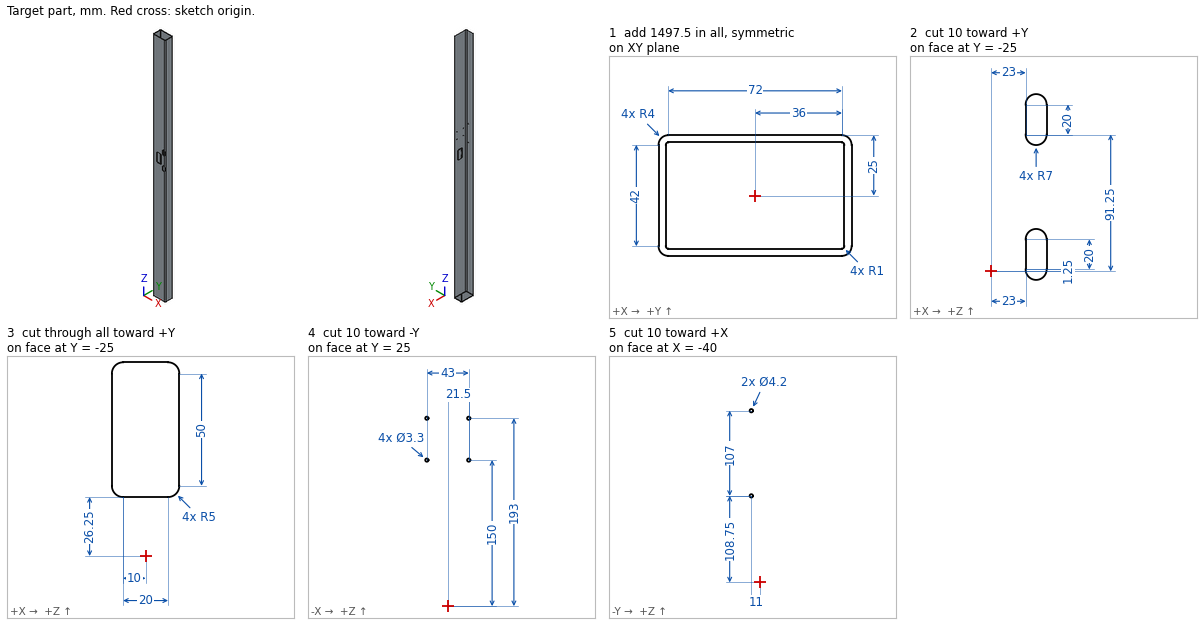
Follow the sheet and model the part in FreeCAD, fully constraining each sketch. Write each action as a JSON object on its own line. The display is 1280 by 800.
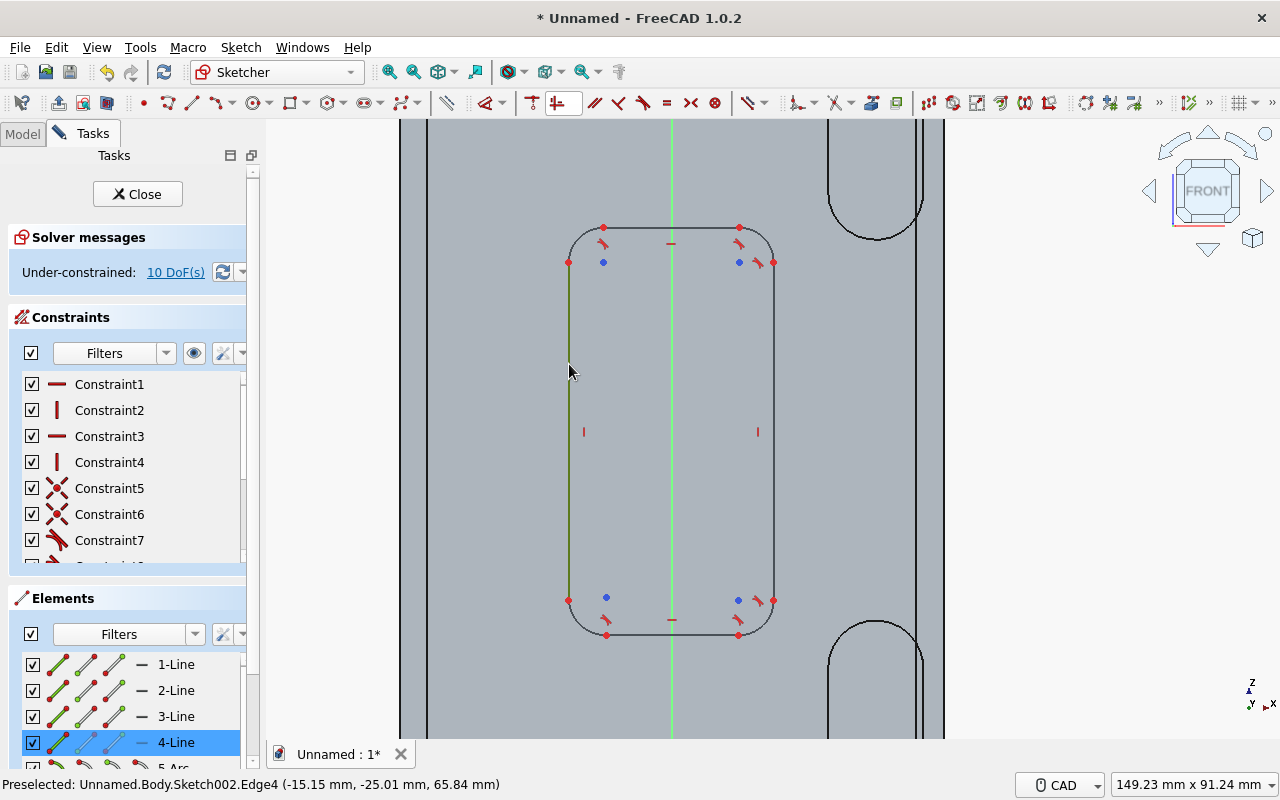
{"action": "left_click", "coordinate": [588, 232]}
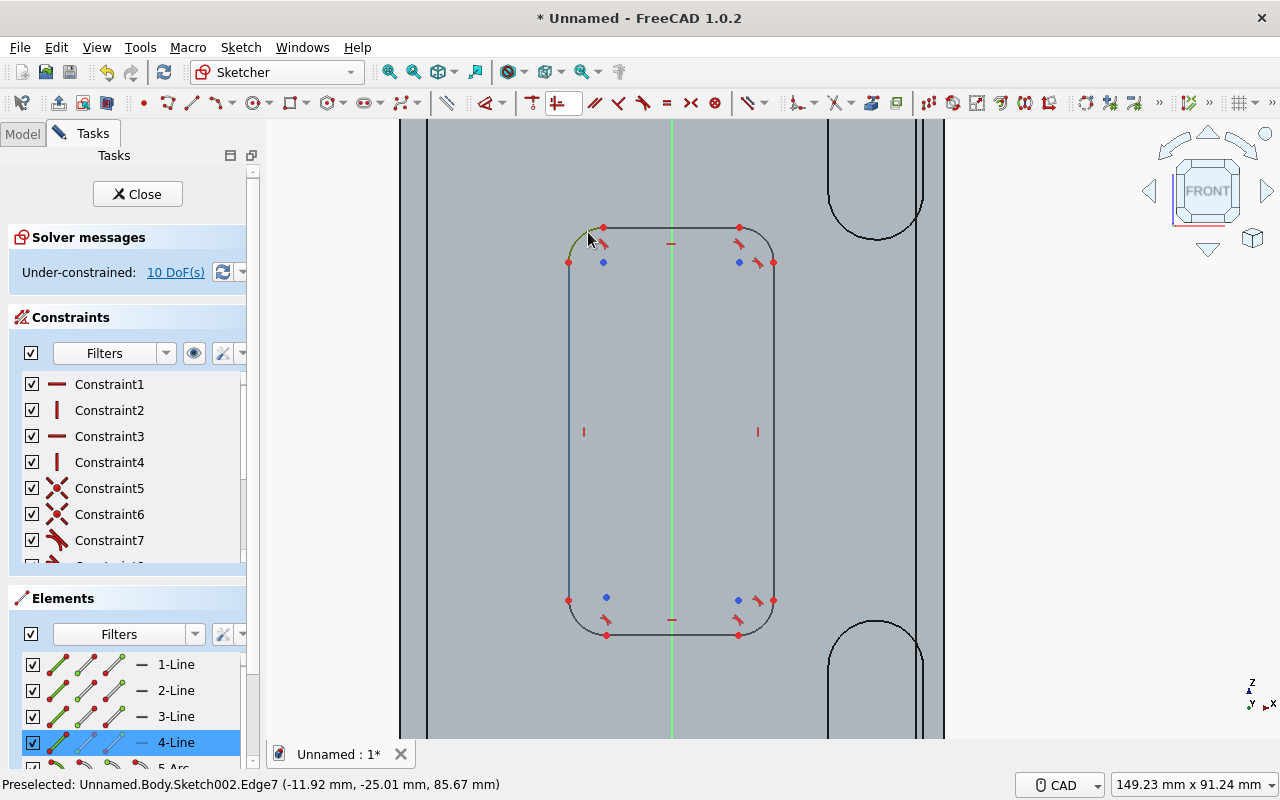
{"action": "key", "text": "t"}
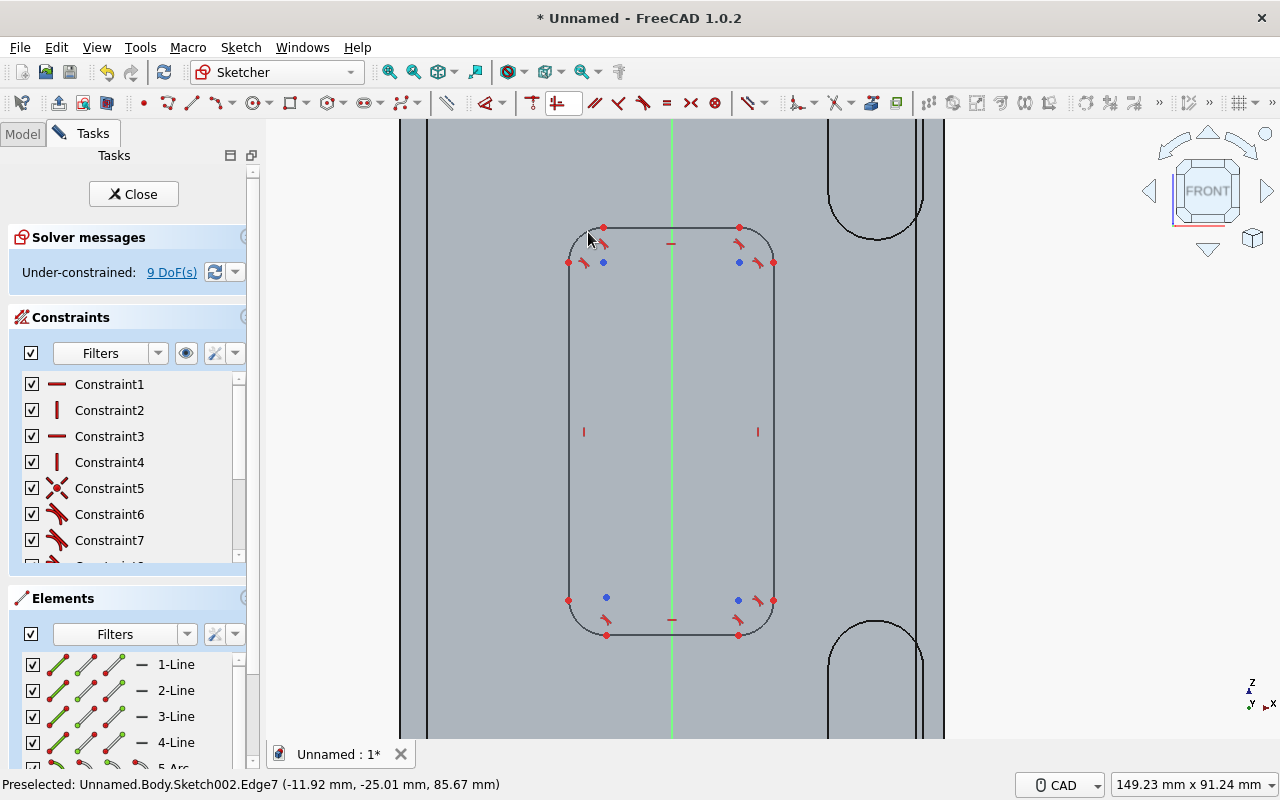
{"action": "left_click", "coordinate": [569, 364]}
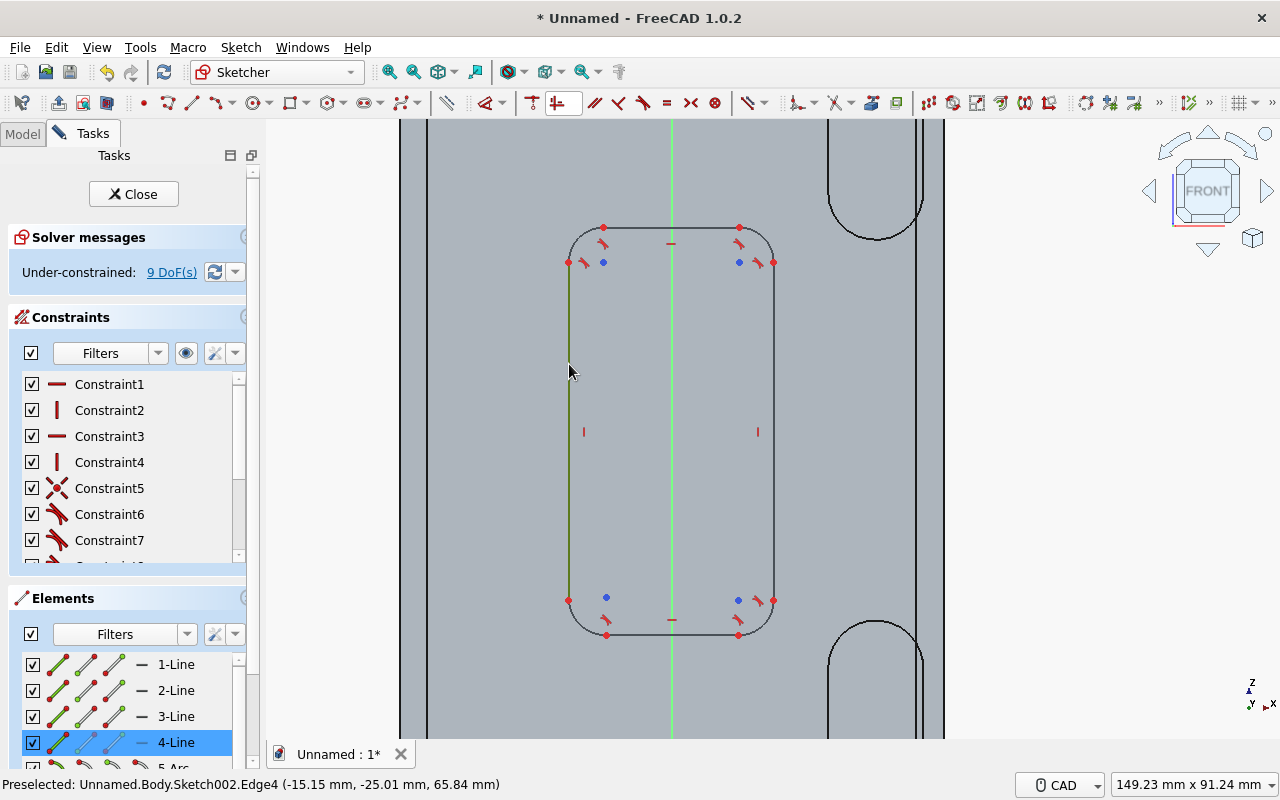
{"action": "left_click", "coordinate": [574, 617]}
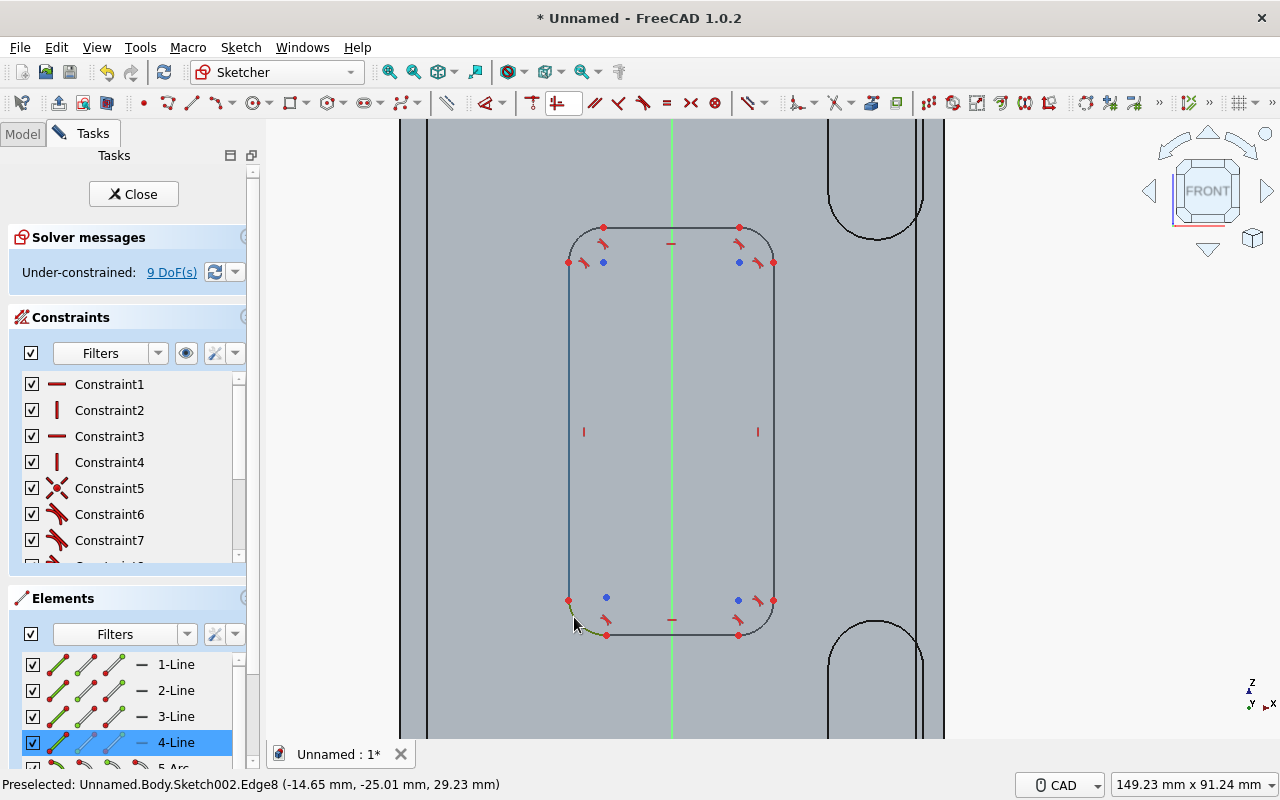
{"action": "left_click", "coordinate": [644, 104]}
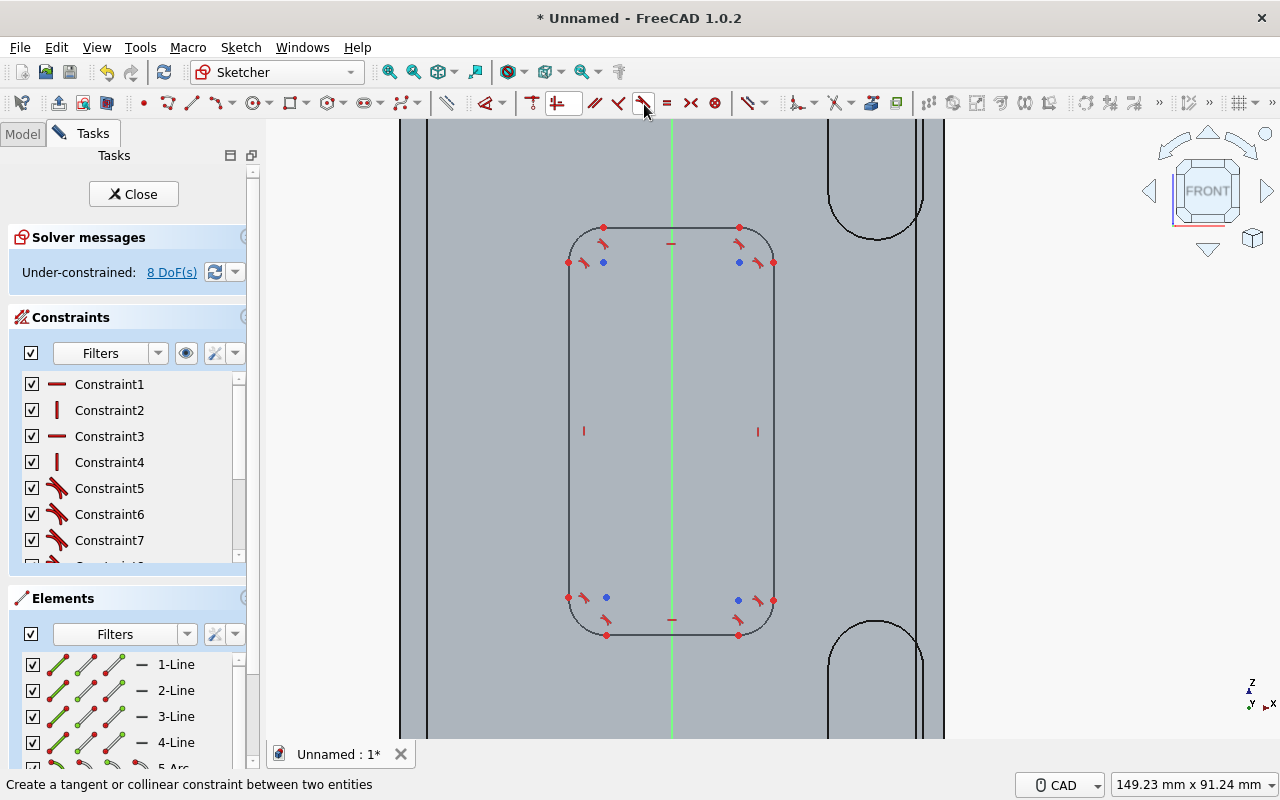
{"action": "left_click", "coordinate": [755, 631]}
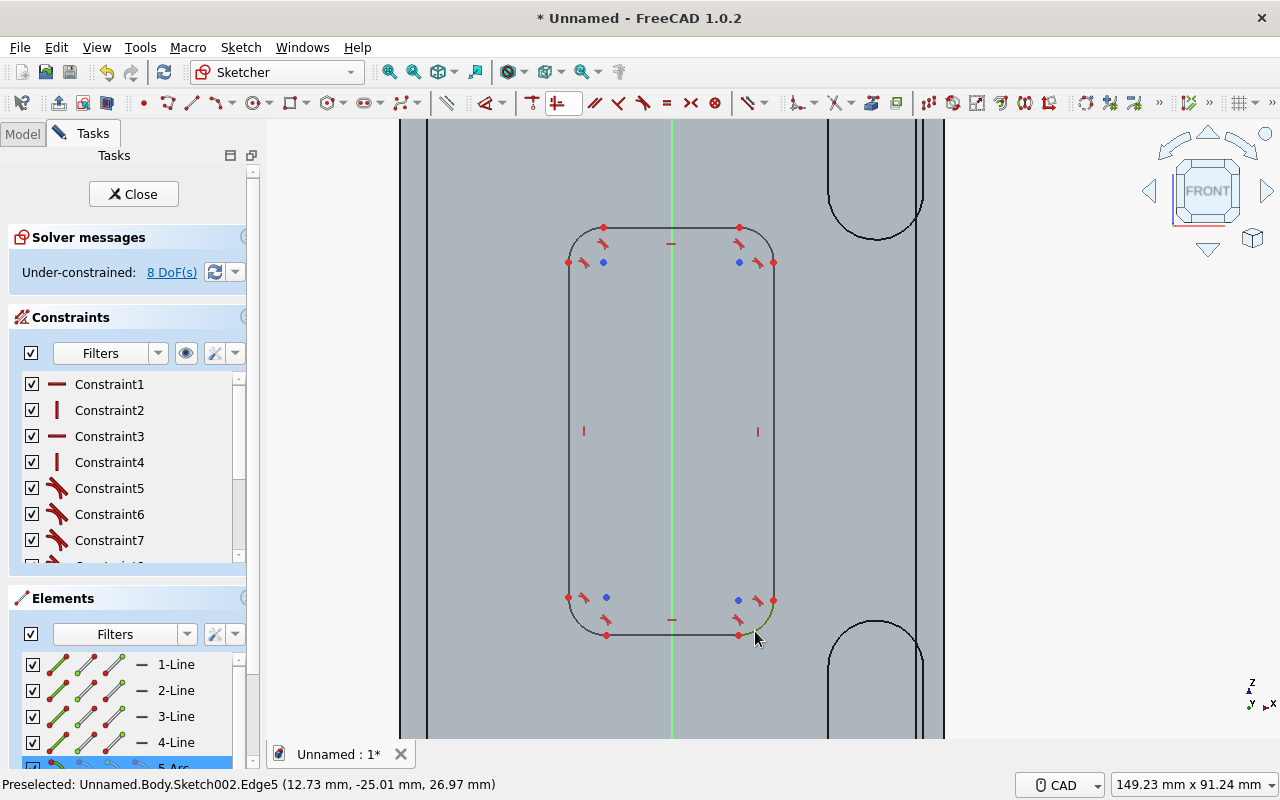
{"action": "left_click", "coordinate": [770, 246]}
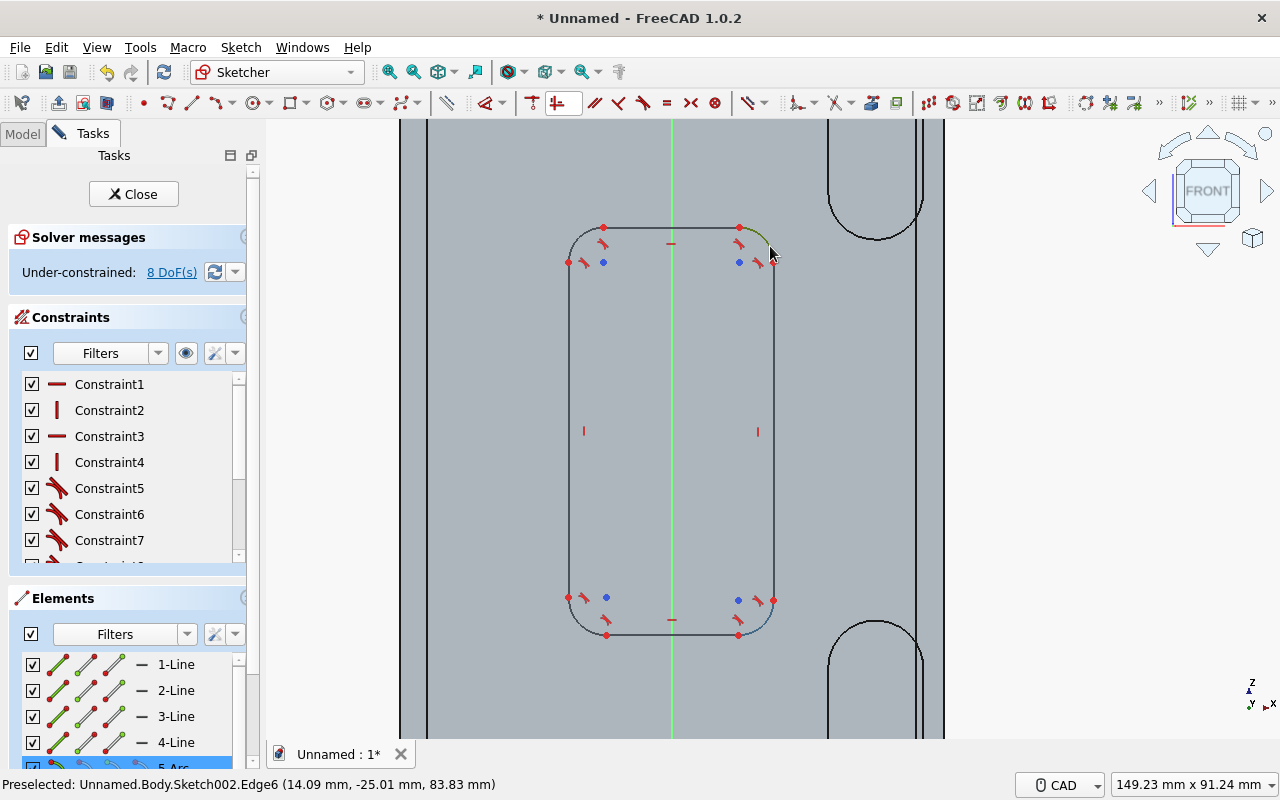
{"action": "left_click", "coordinate": [588, 231]}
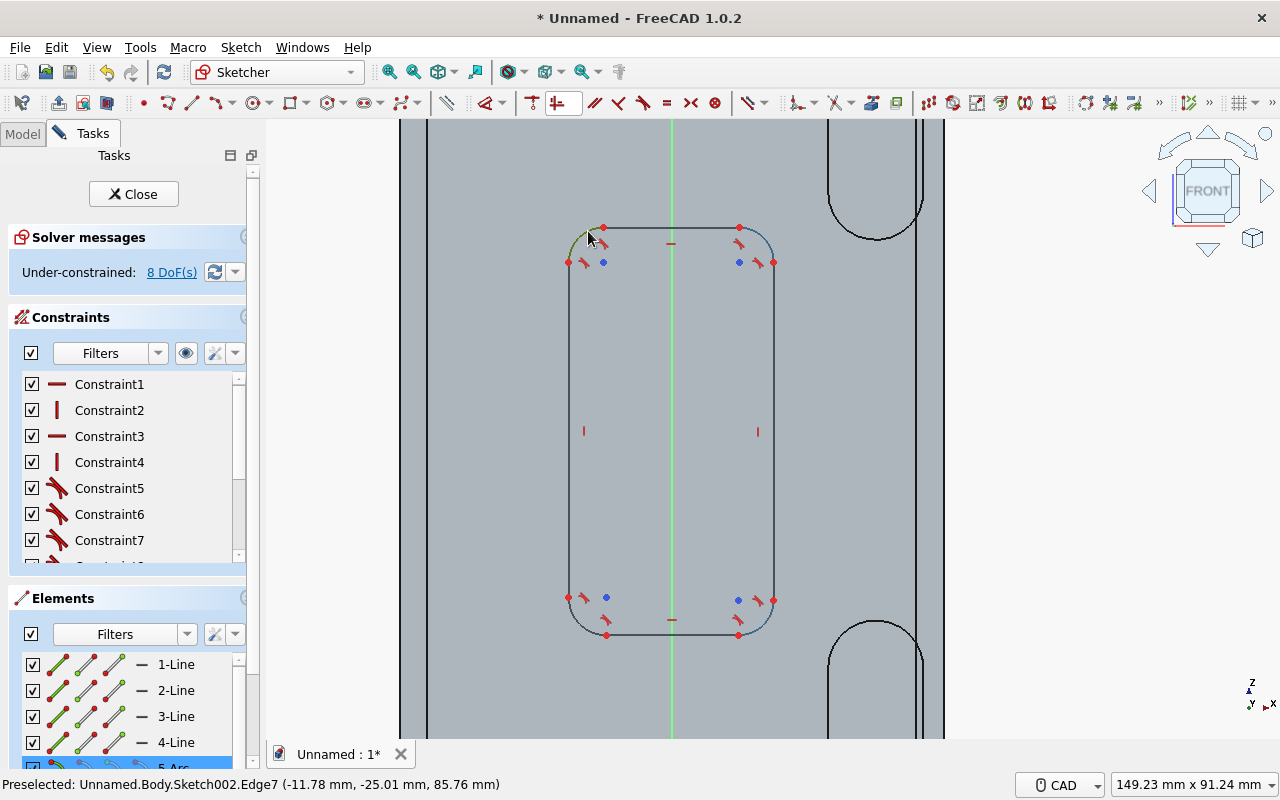
{"action": "left_click", "coordinate": [573, 615]}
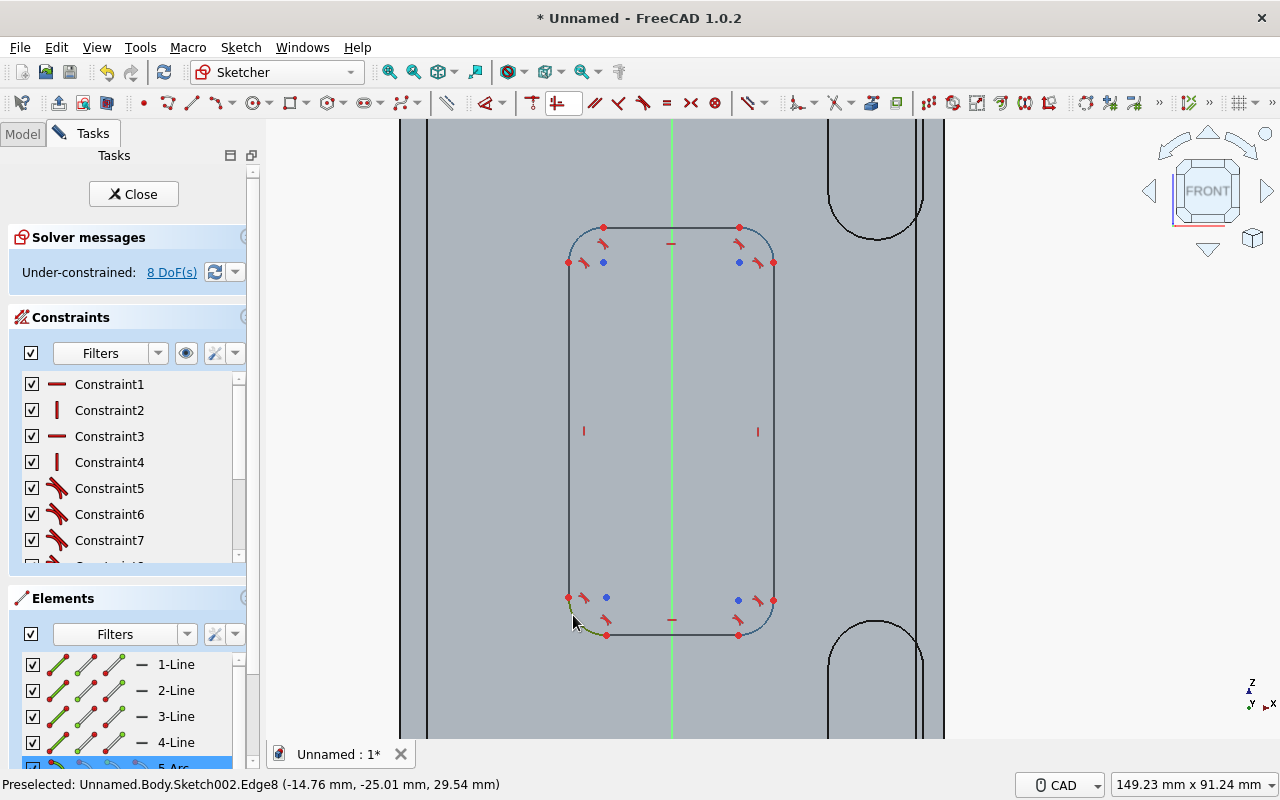
{"action": "left_click", "coordinate": [668, 104]}